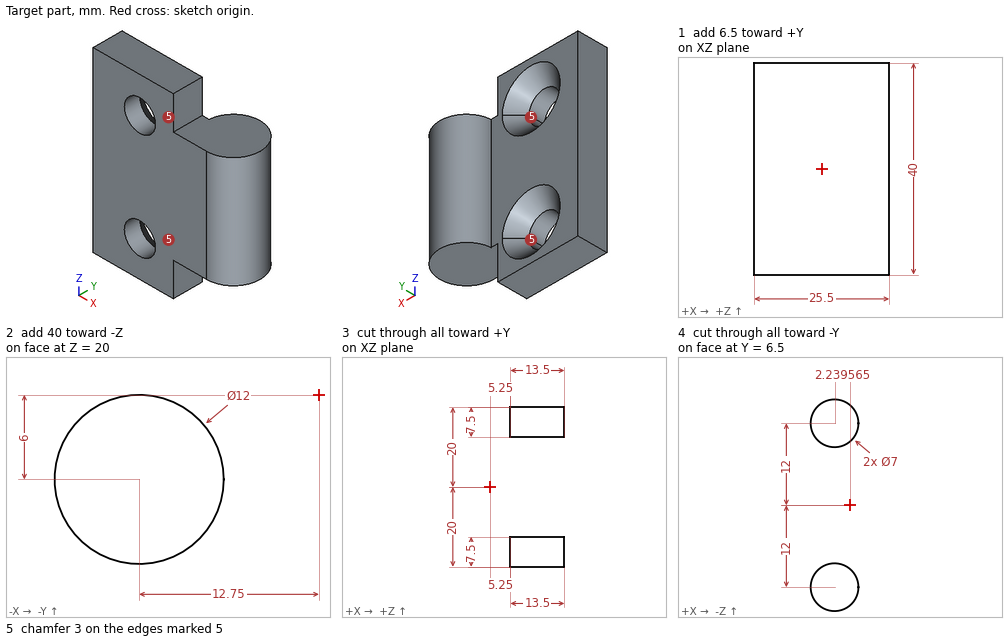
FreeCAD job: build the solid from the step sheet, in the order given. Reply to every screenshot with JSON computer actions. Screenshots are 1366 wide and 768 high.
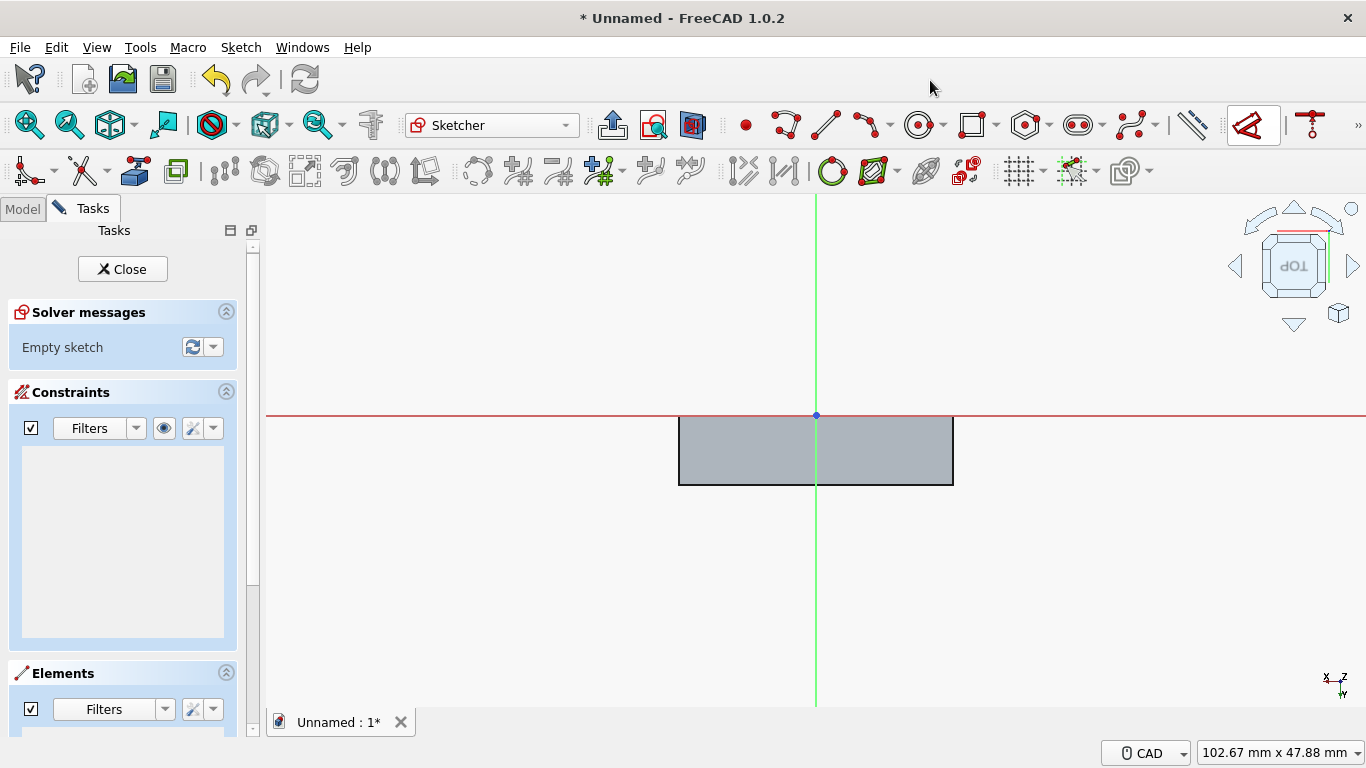
{"action": "scroll", "coordinate": [697, 497], "scroll_direction": "up", "scroll_amount": 5}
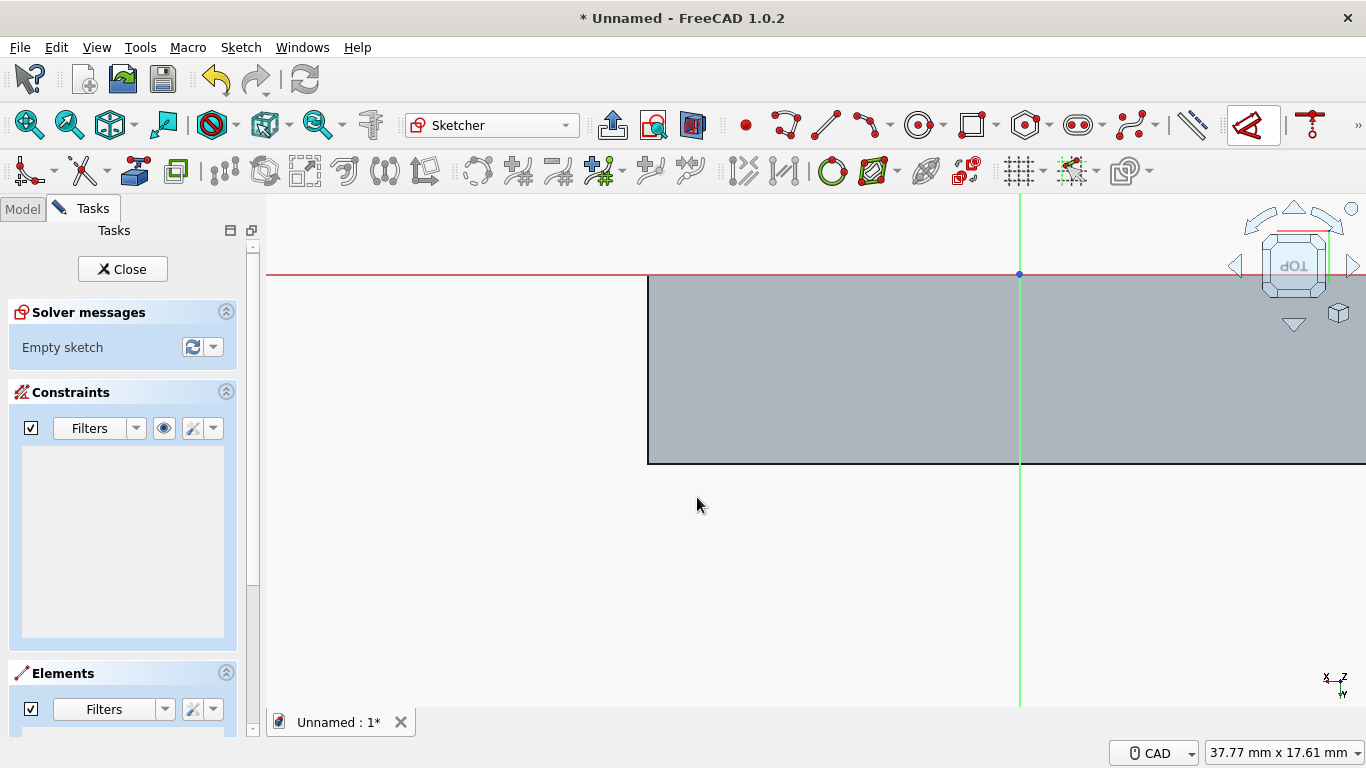
{"action": "left_click", "coordinate": [920, 126]}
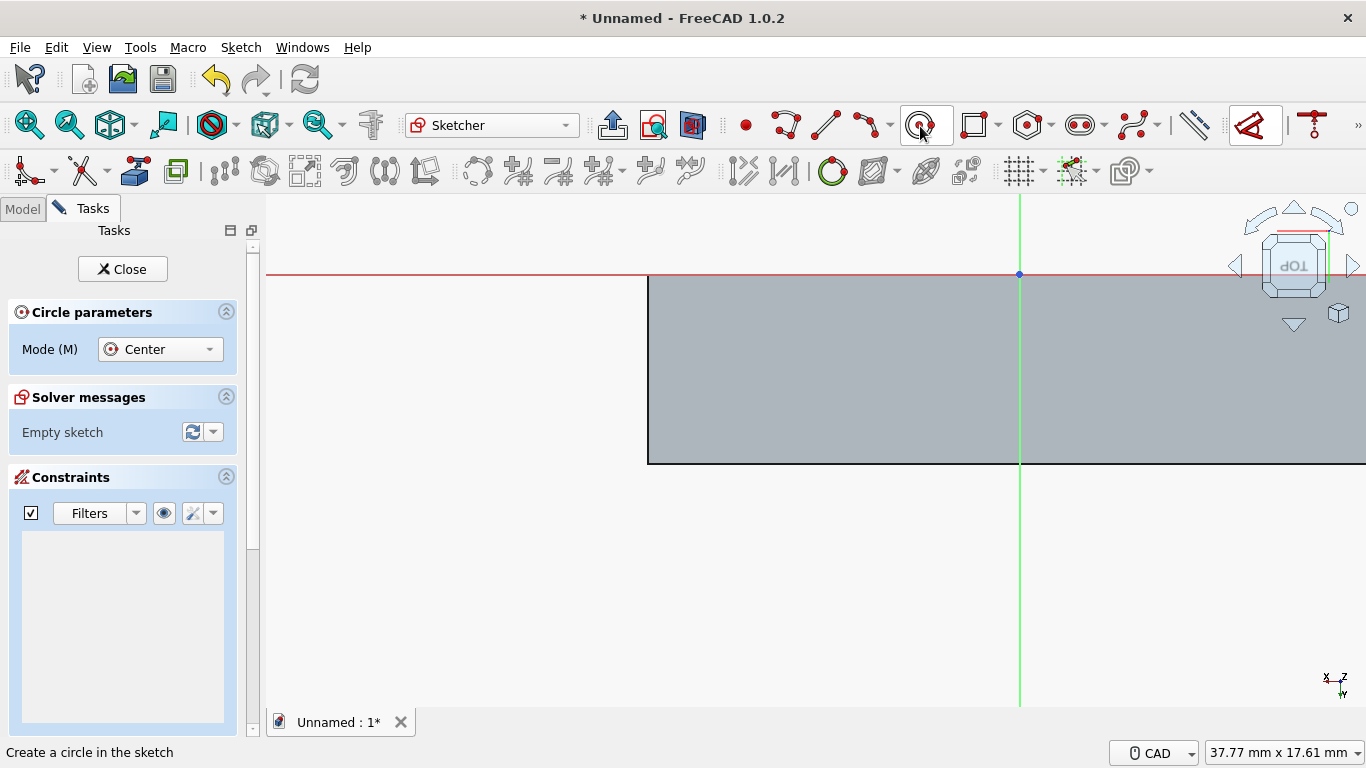
{"action": "left_click", "coordinate": [648, 450]}
{"action": "left_click", "coordinate": [772, 326]}
{"action": "key", "text": "Escape"}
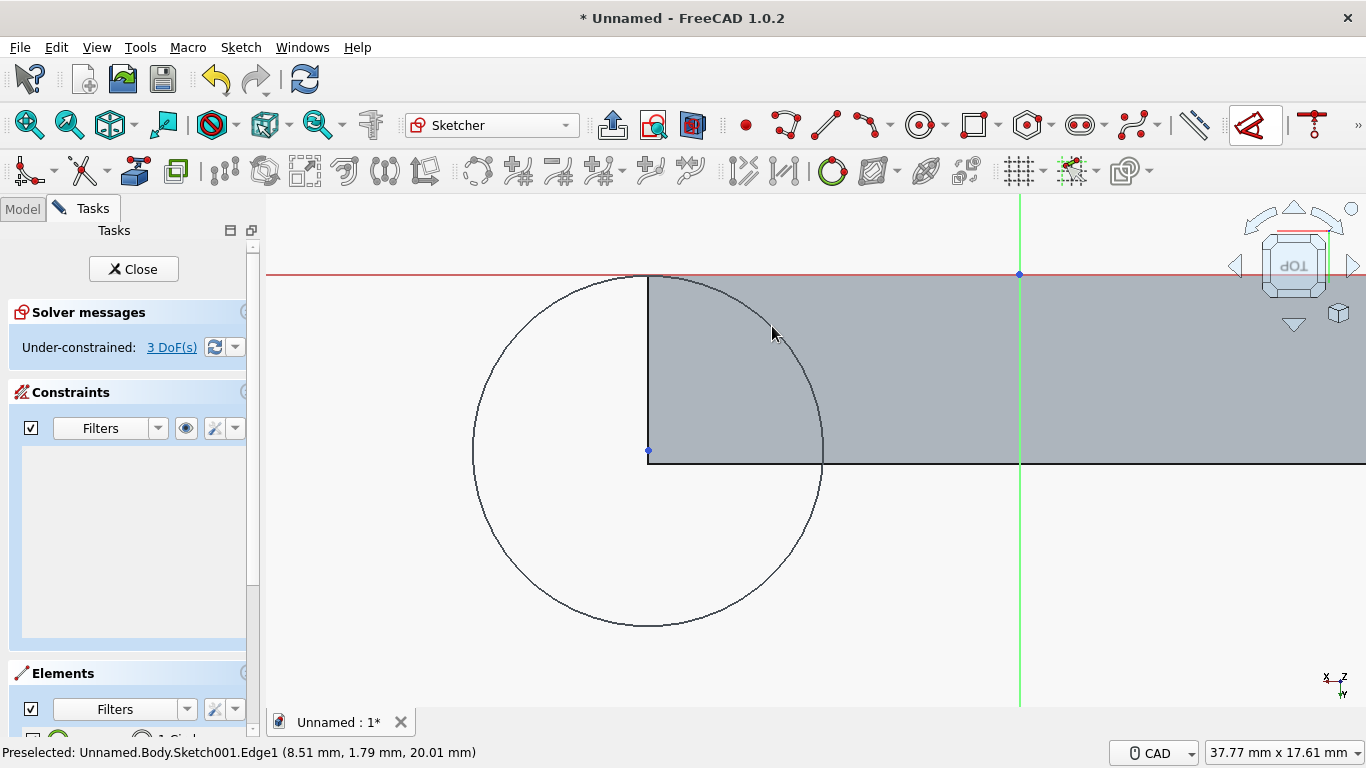
{"action": "left_click", "coordinate": [1250, 126]}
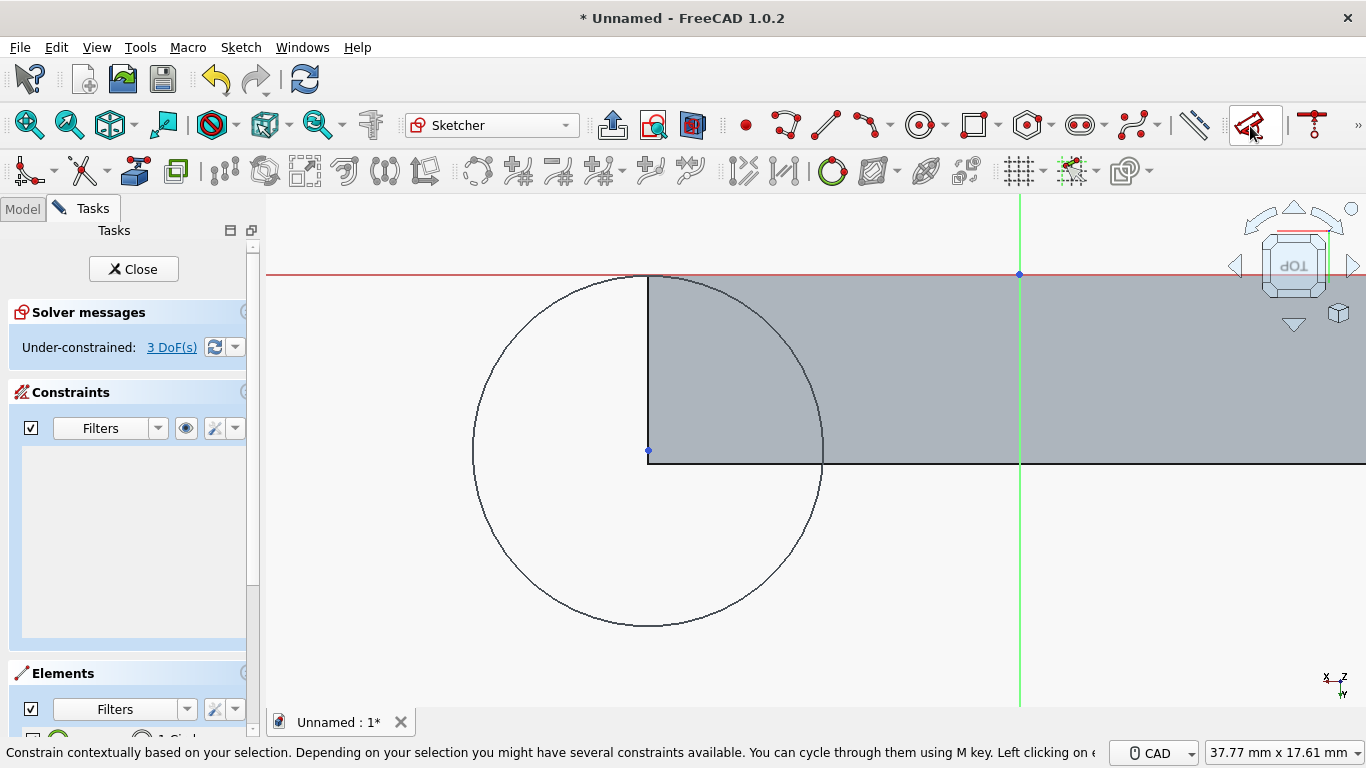
{"action": "left_click", "coordinate": [772, 327]}
{"action": "left_click", "coordinate": [795, 304]}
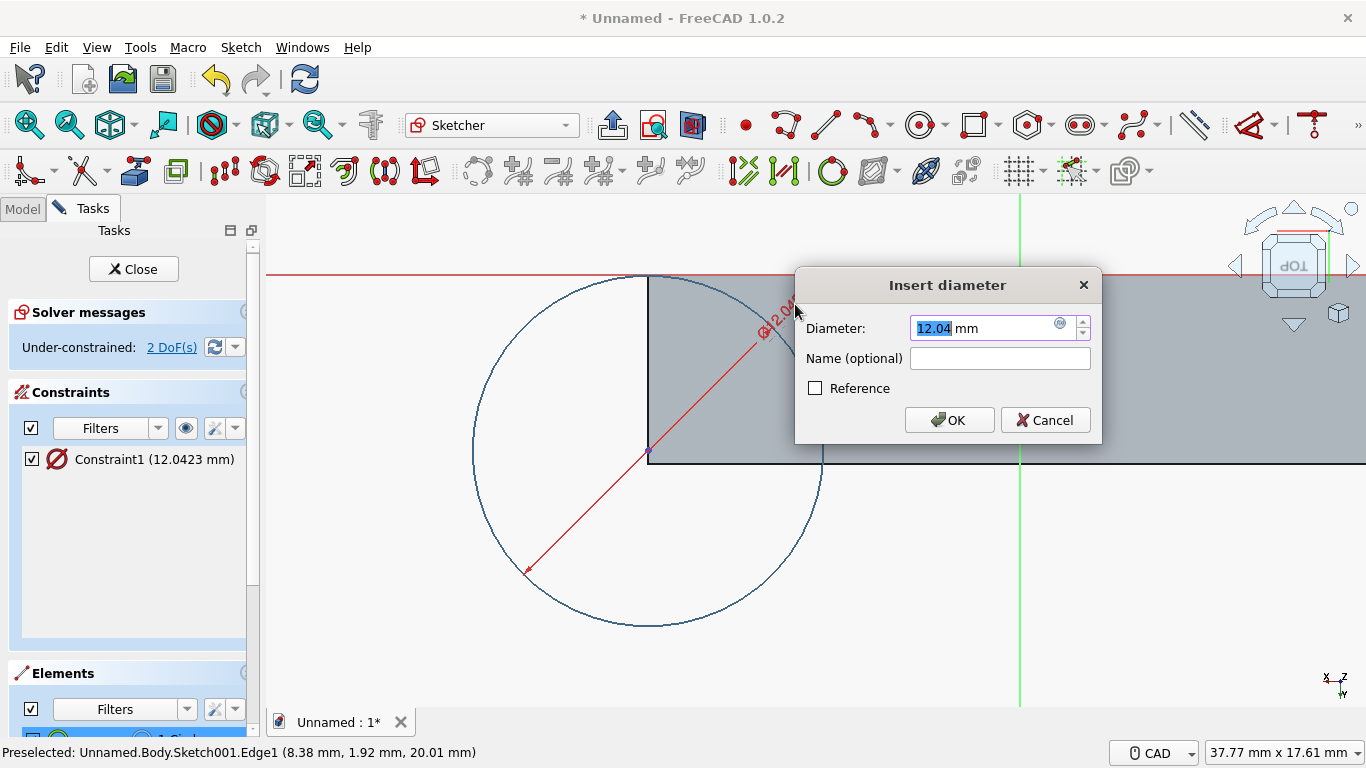
{"action": "type", "text": "12"}
{"action": "key", "text": "Return"}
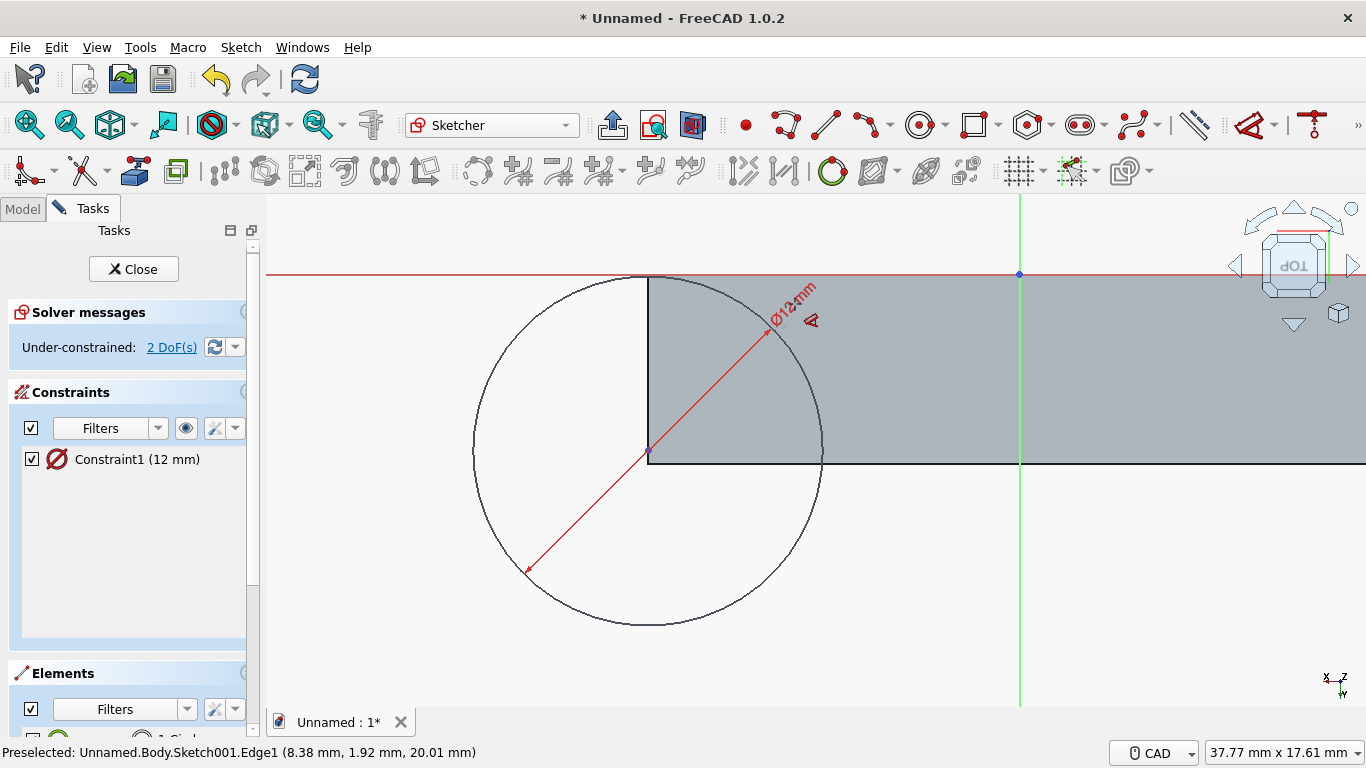
{"action": "left_click", "coordinate": [648, 451]}
{"action": "left_click", "coordinate": [1054, 363]}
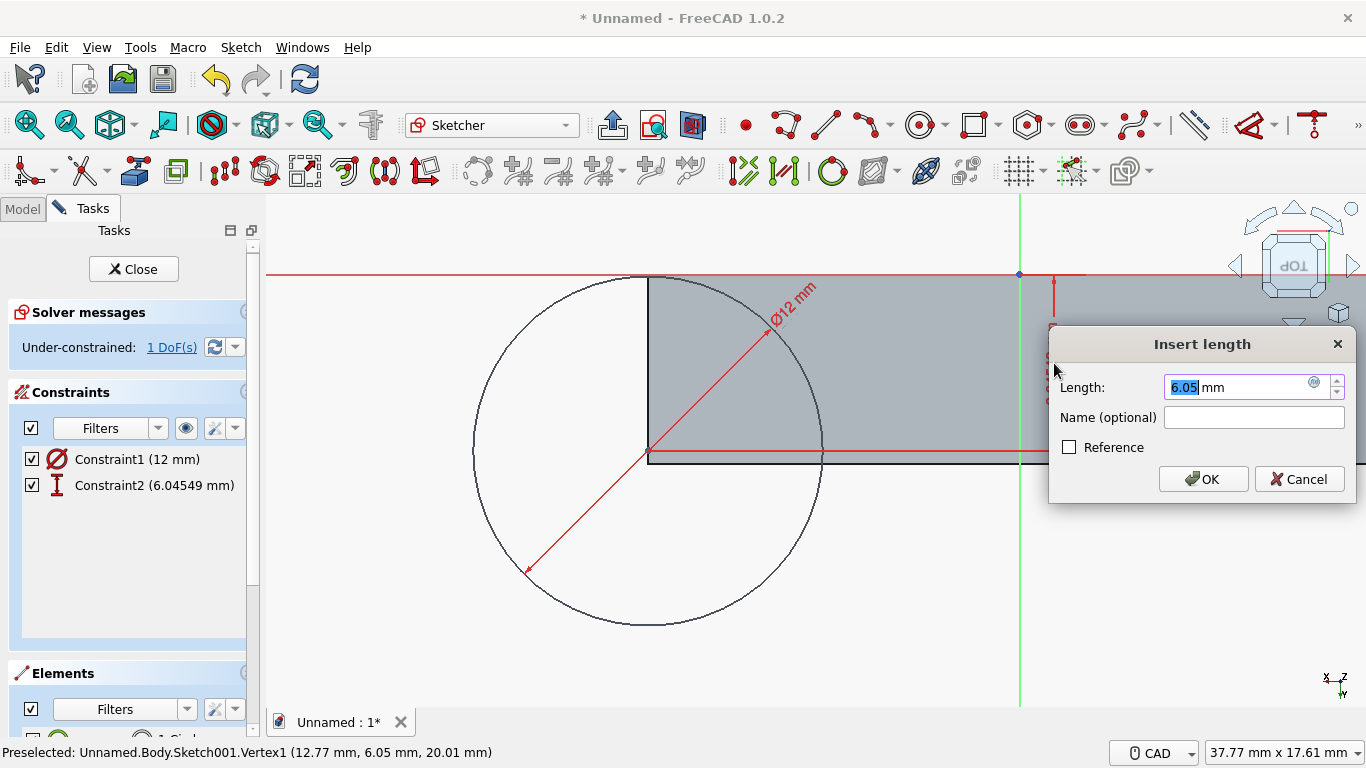
{"action": "type", "text": "6"}
{"action": "key", "text": "Return"}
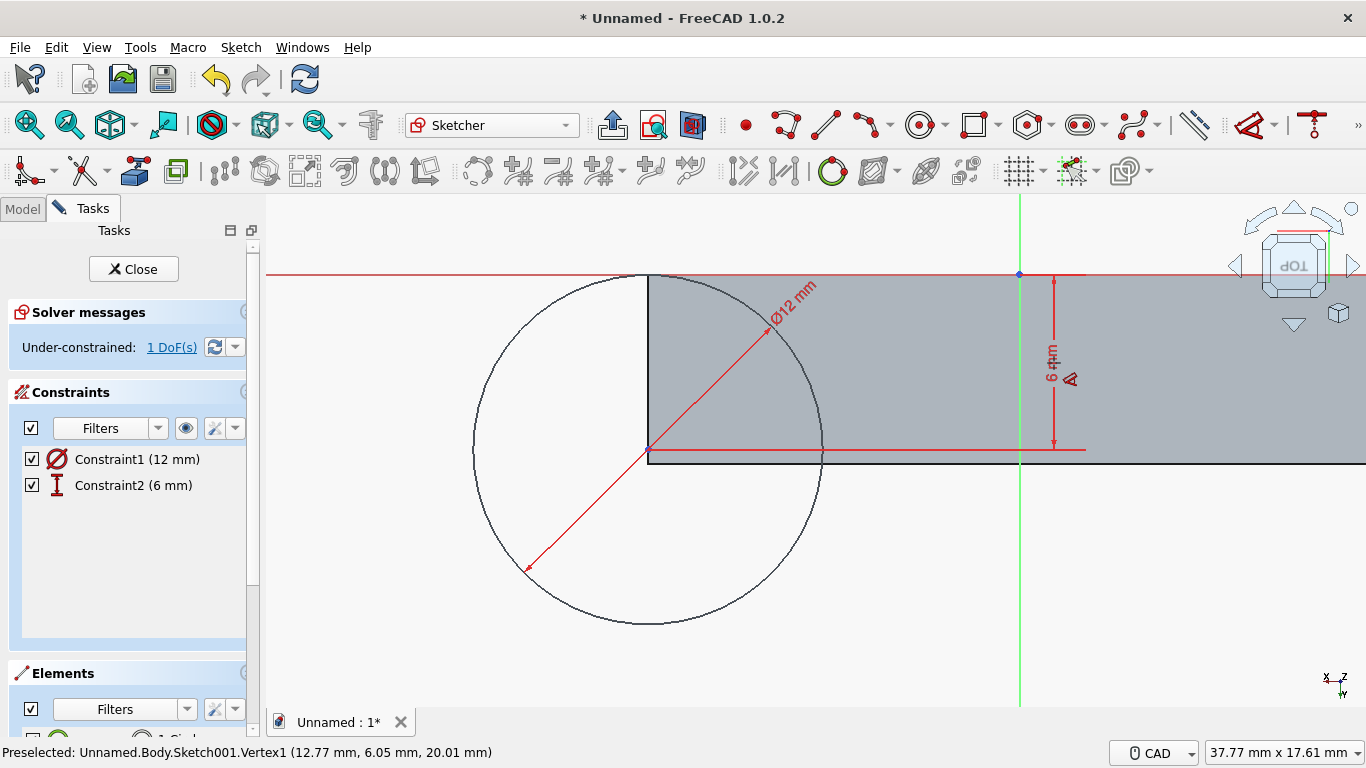
{"action": "left_click", "coordinate": [648, 450]}
{"action": "left_click", "coordinate": [834, 241]}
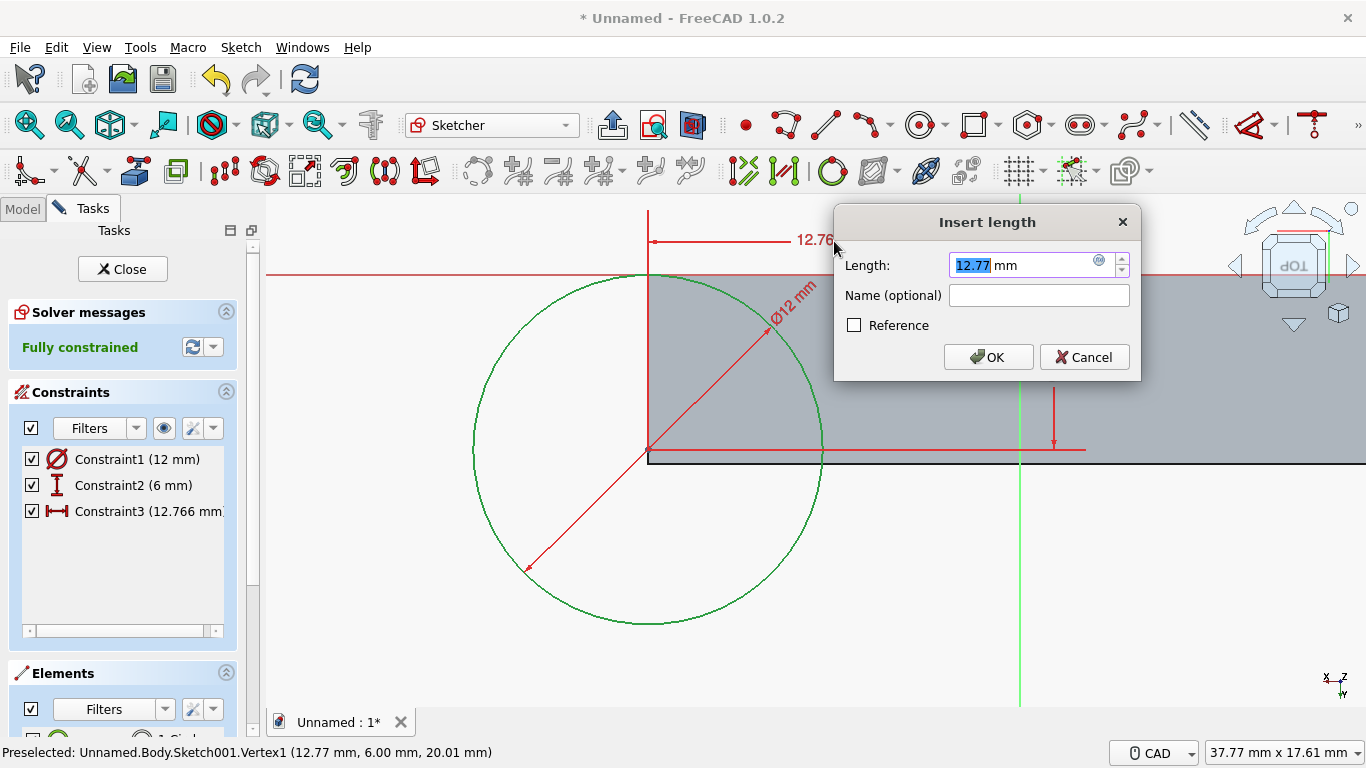
{"action": "type", "text": "12.75"}
{"action": "key", "text": "Return"}
{"action": "key", "text": "Escape"}